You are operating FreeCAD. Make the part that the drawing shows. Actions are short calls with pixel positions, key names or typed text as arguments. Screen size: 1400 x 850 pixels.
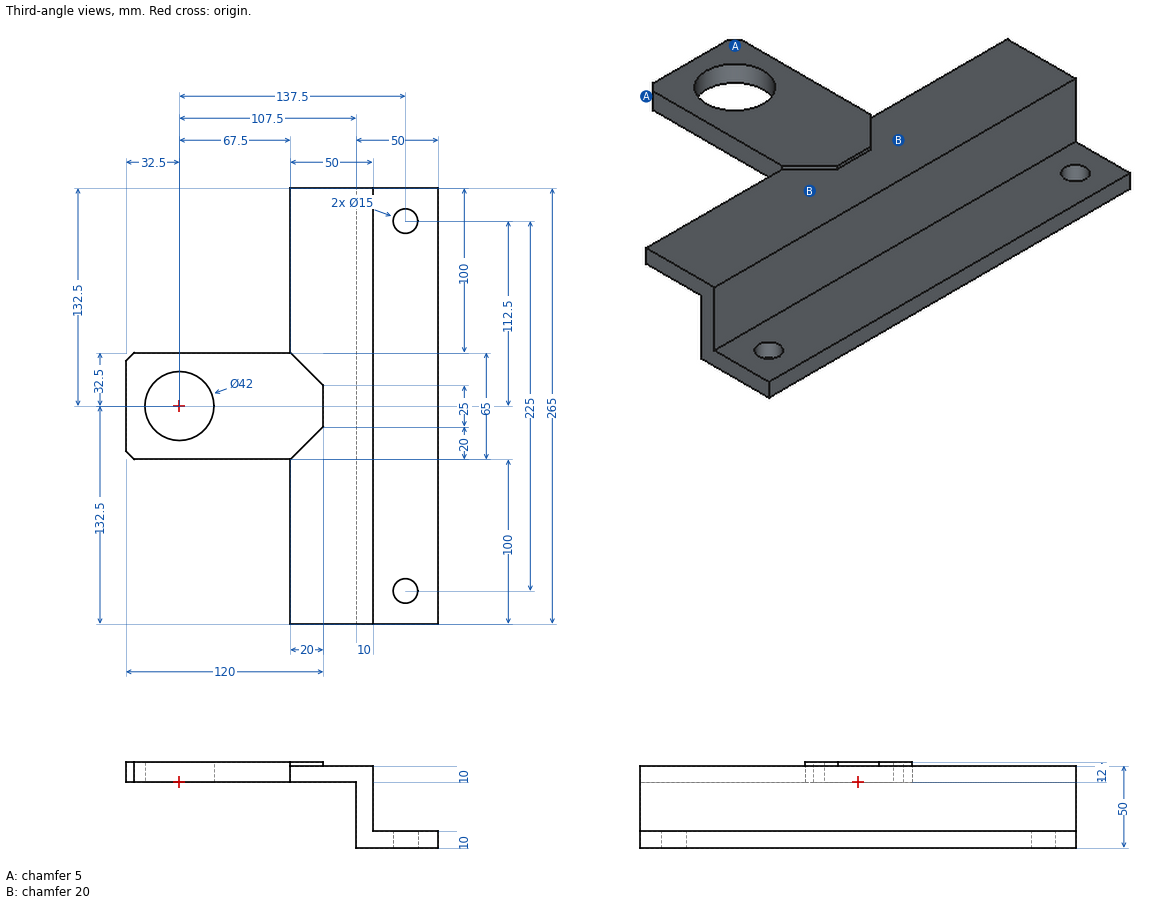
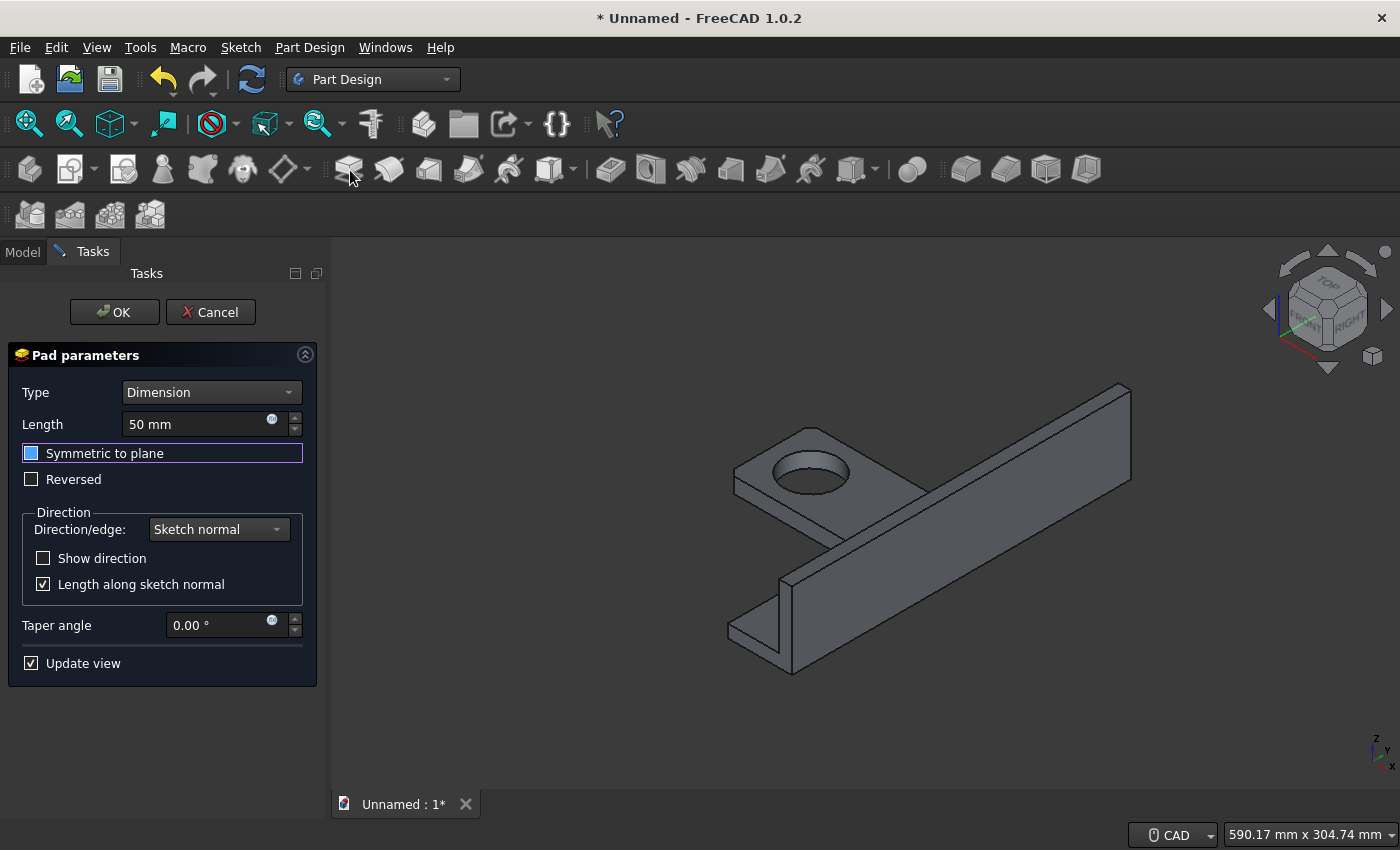
click(30, 479)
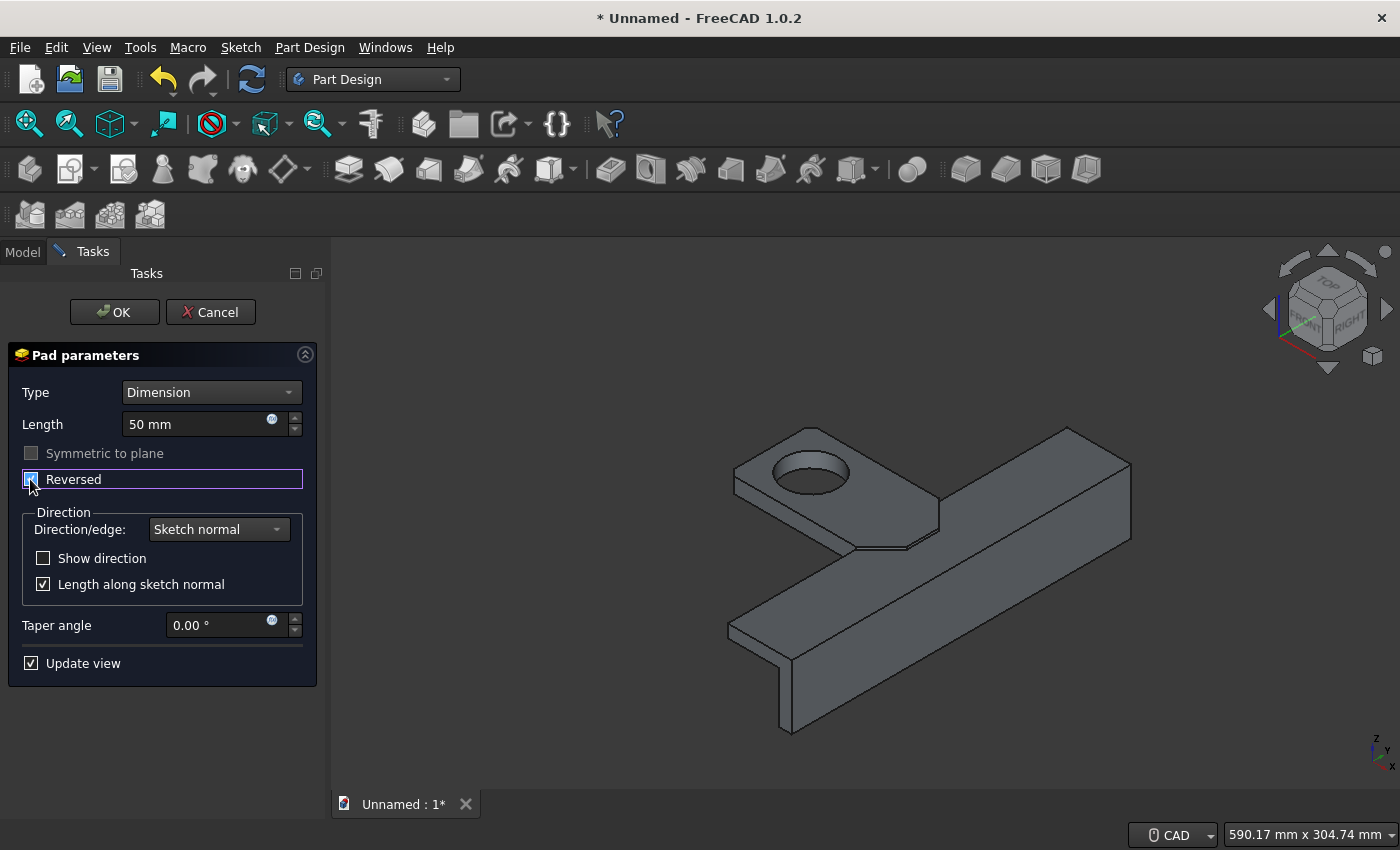
click(115, 312)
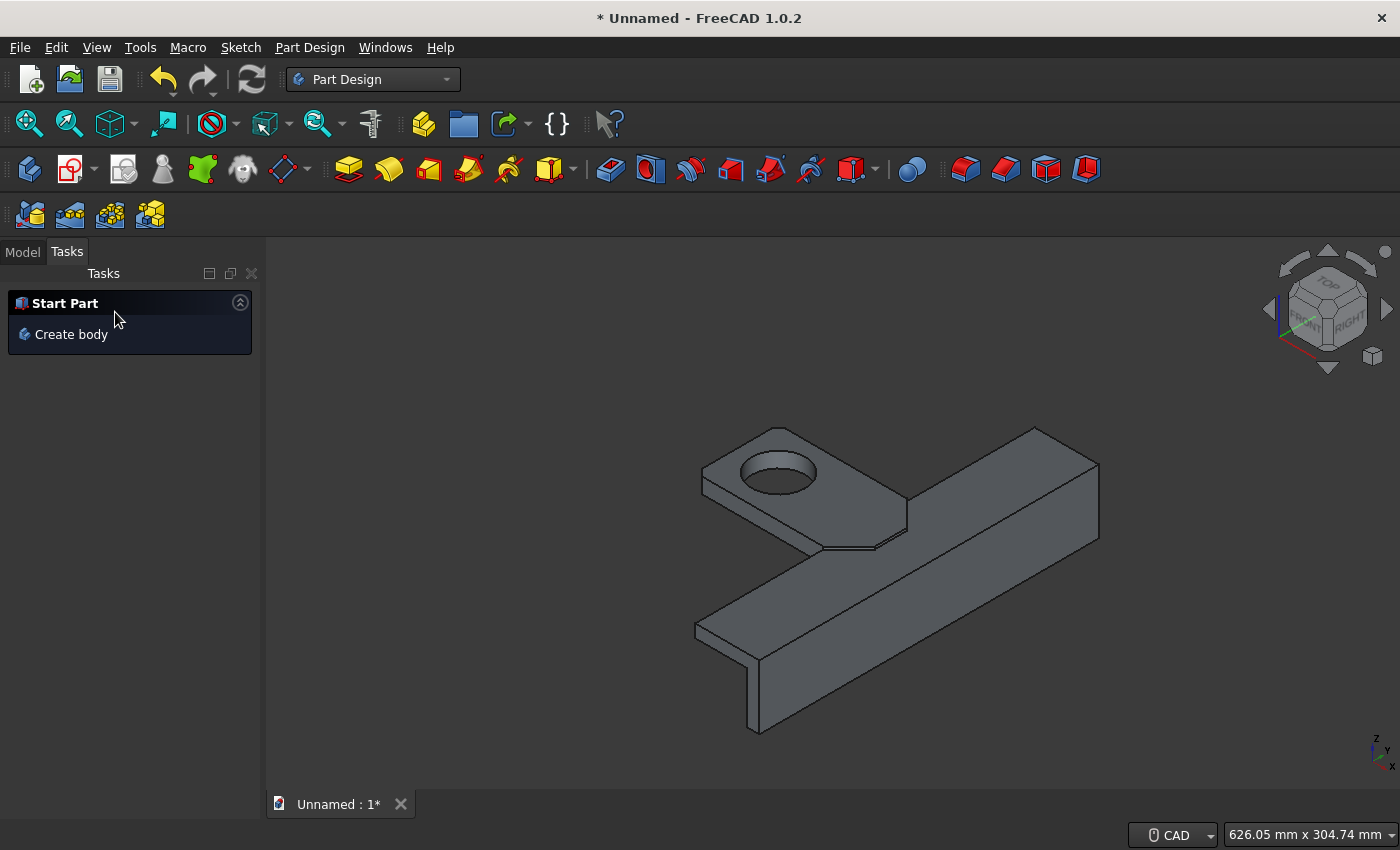
key(5)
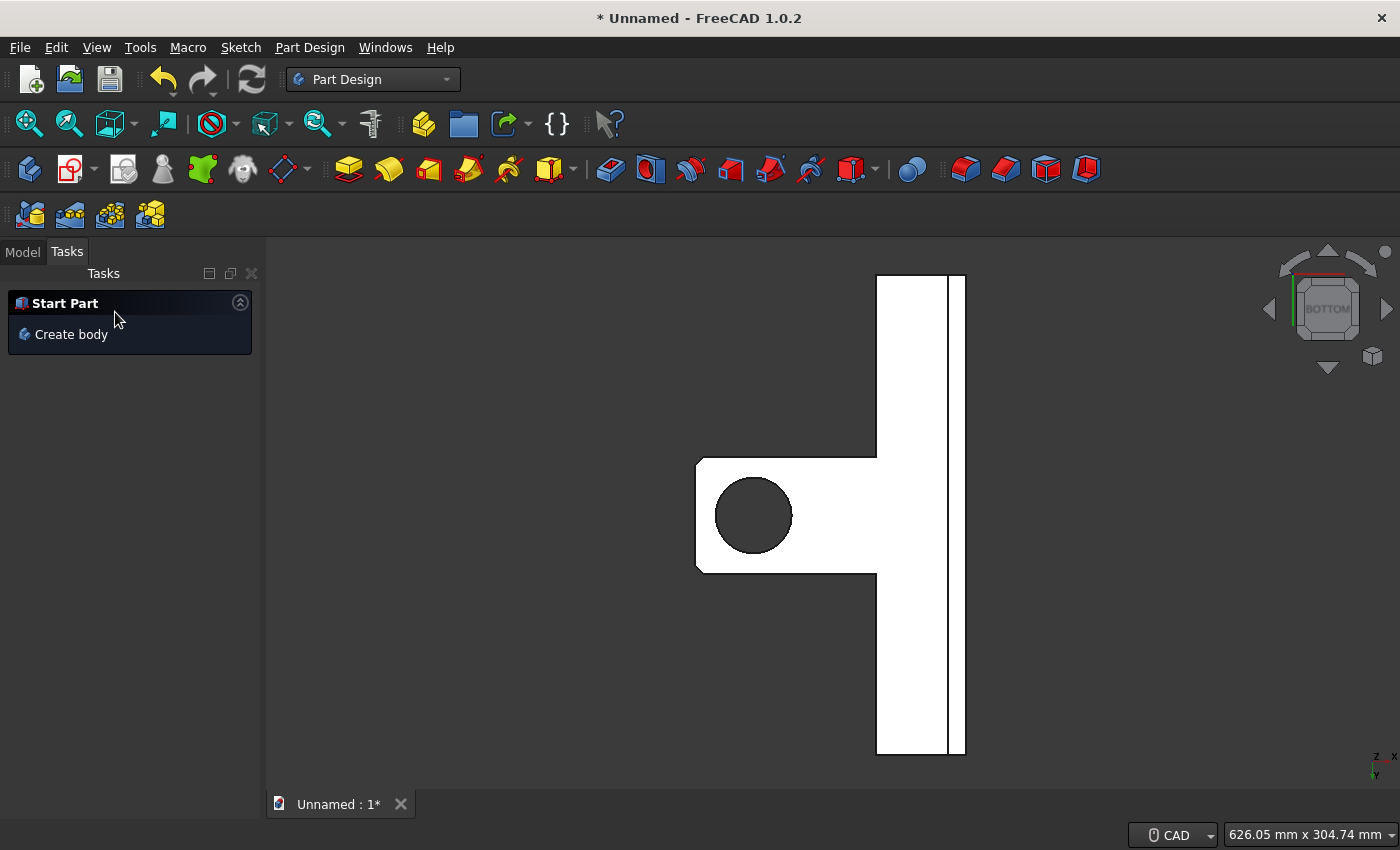
click(957, 720)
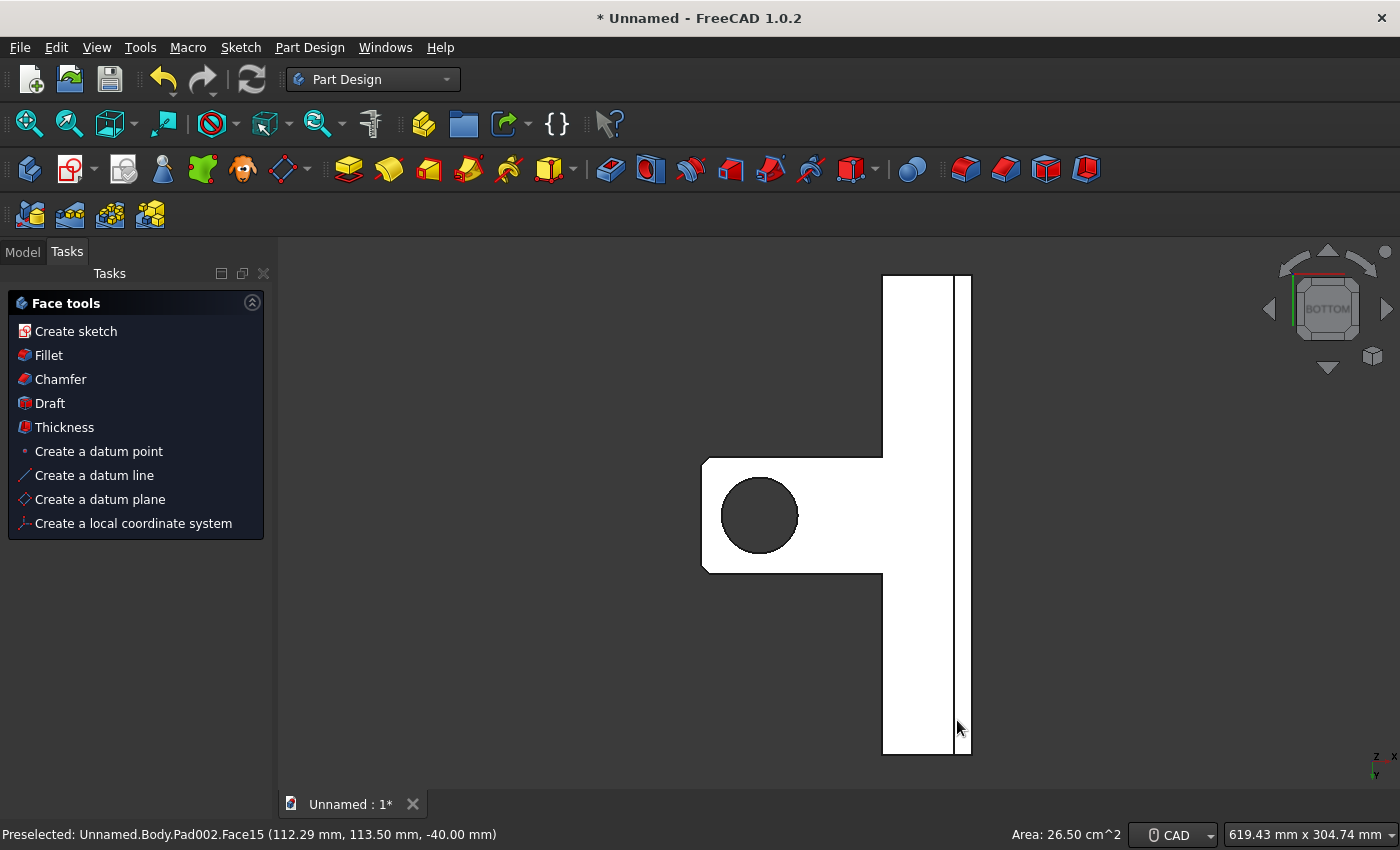
click(70, 170)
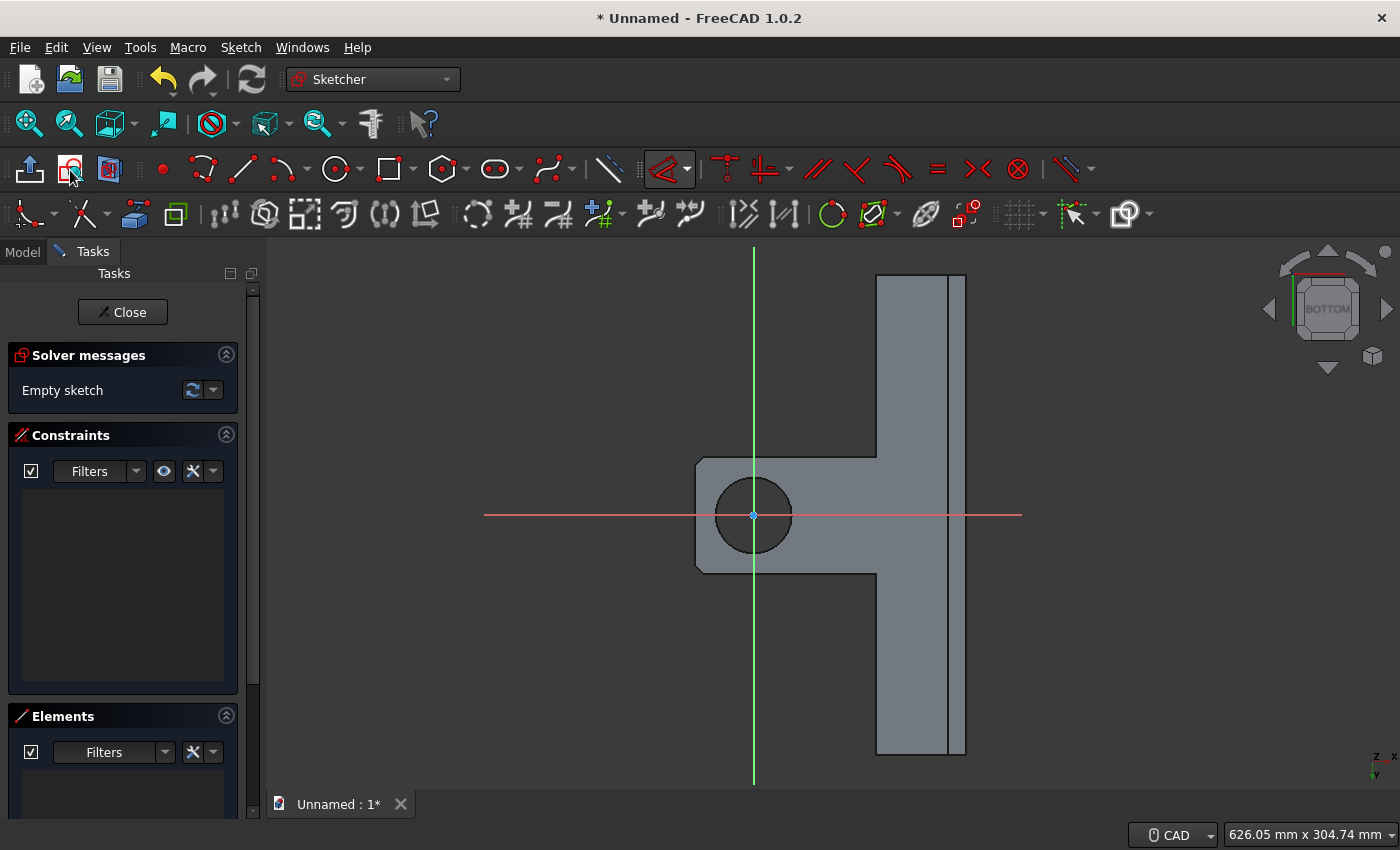
scroll(497, 508, down, 2)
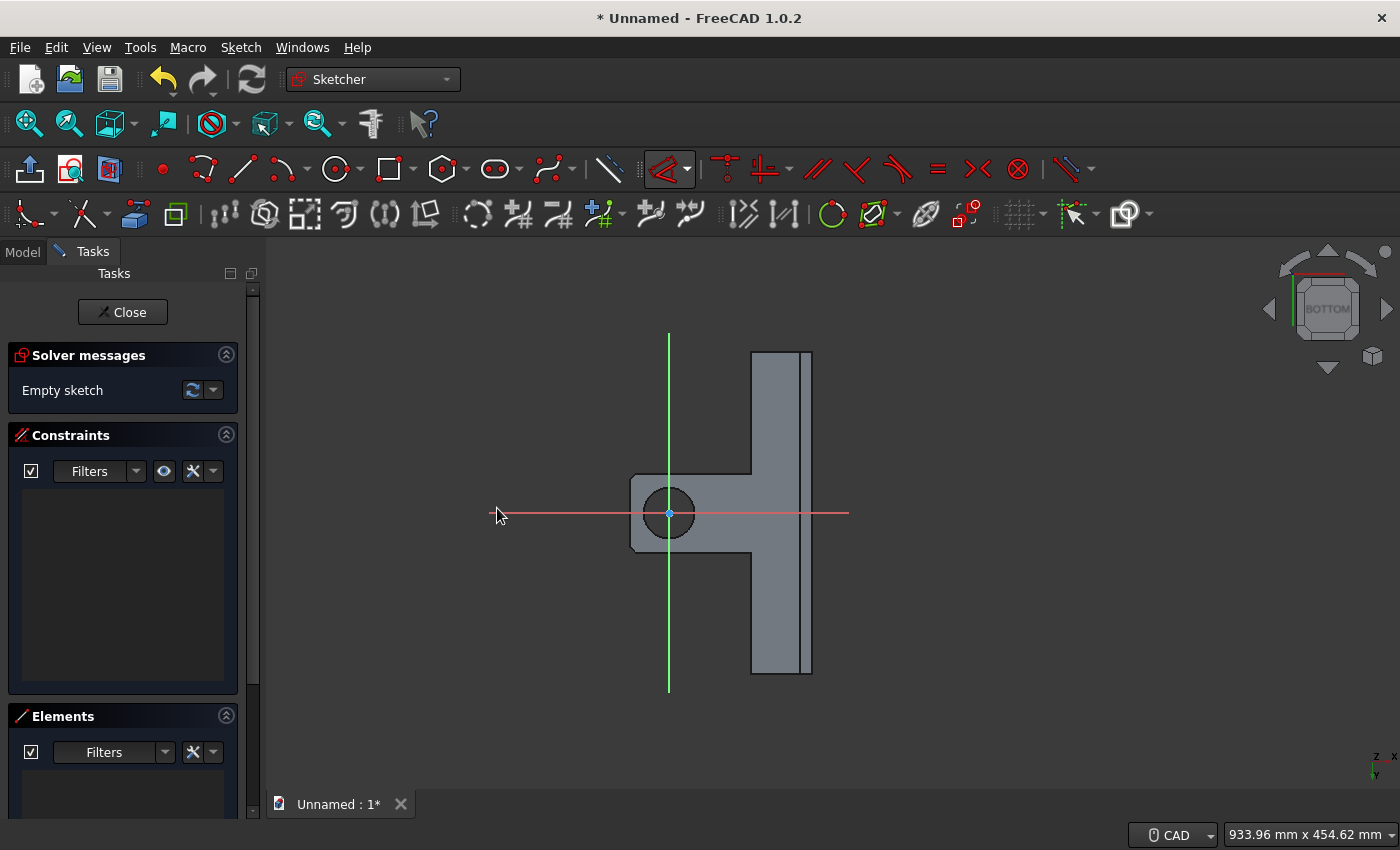
key(g)
key(r)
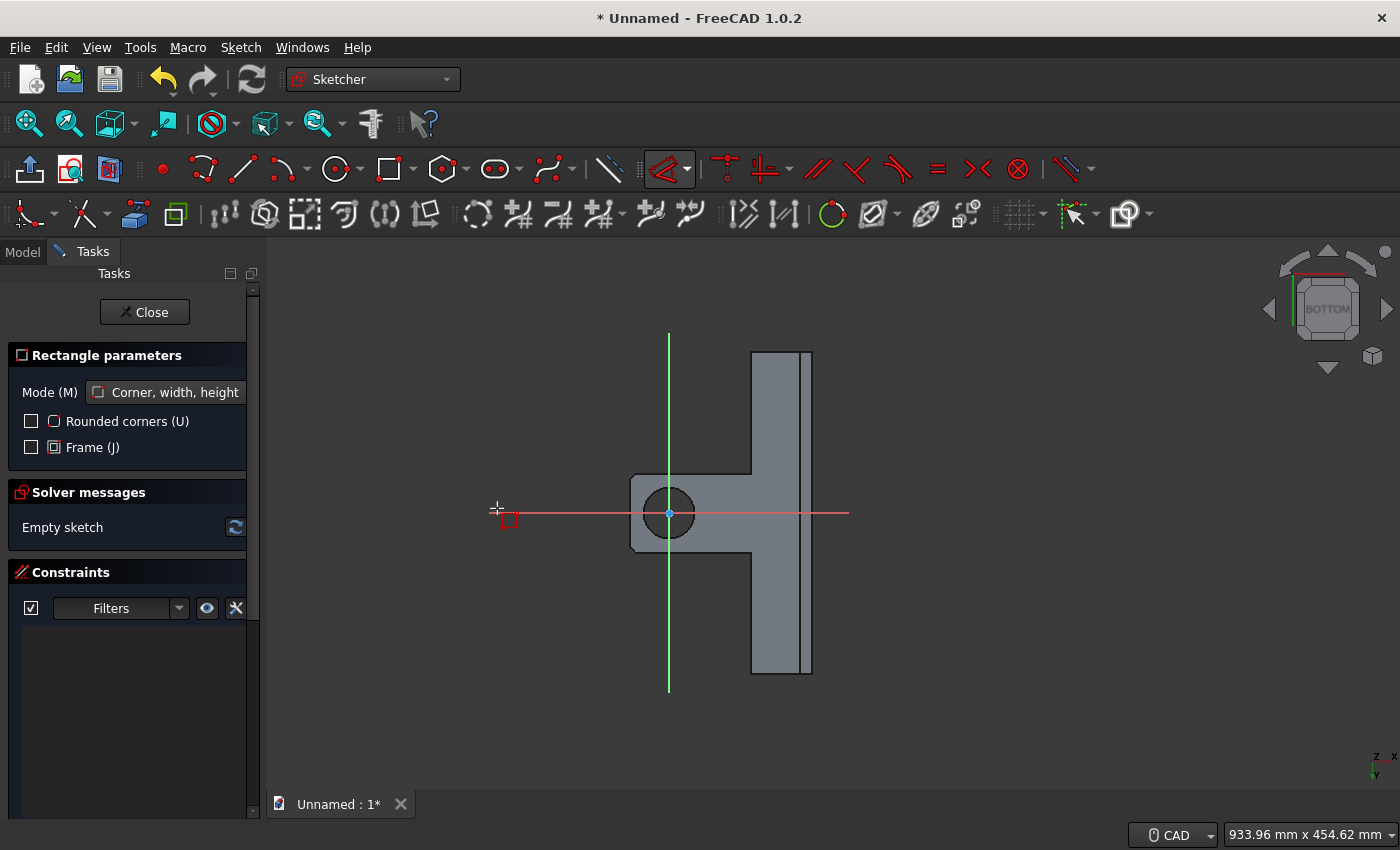
click(800, 352)
move(860, 674)